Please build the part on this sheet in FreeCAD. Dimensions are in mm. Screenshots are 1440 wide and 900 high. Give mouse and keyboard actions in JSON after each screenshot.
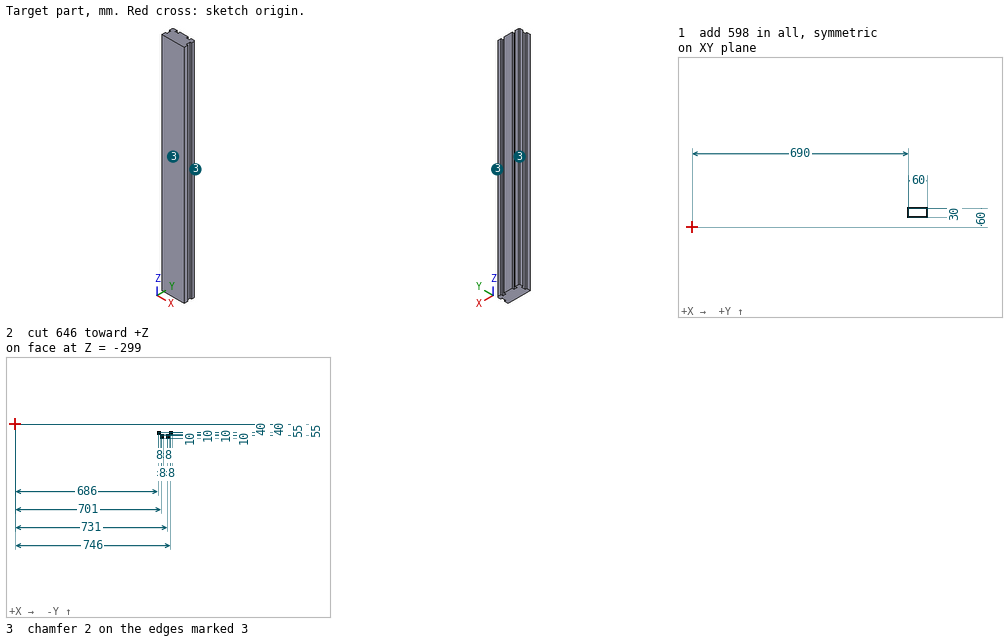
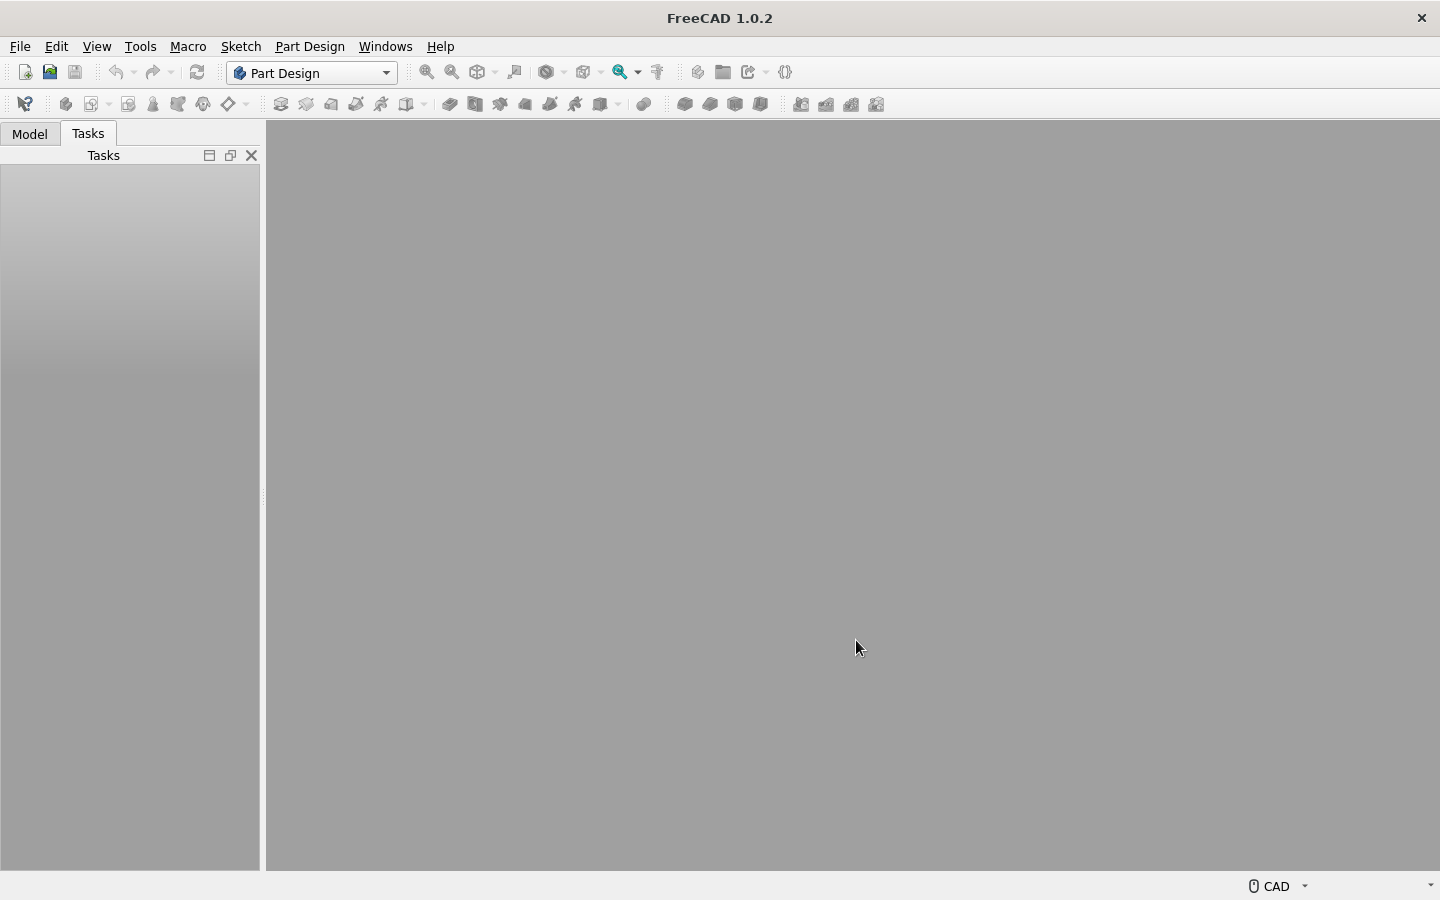
{"action": "left_click", "coordinate": [25, 72]}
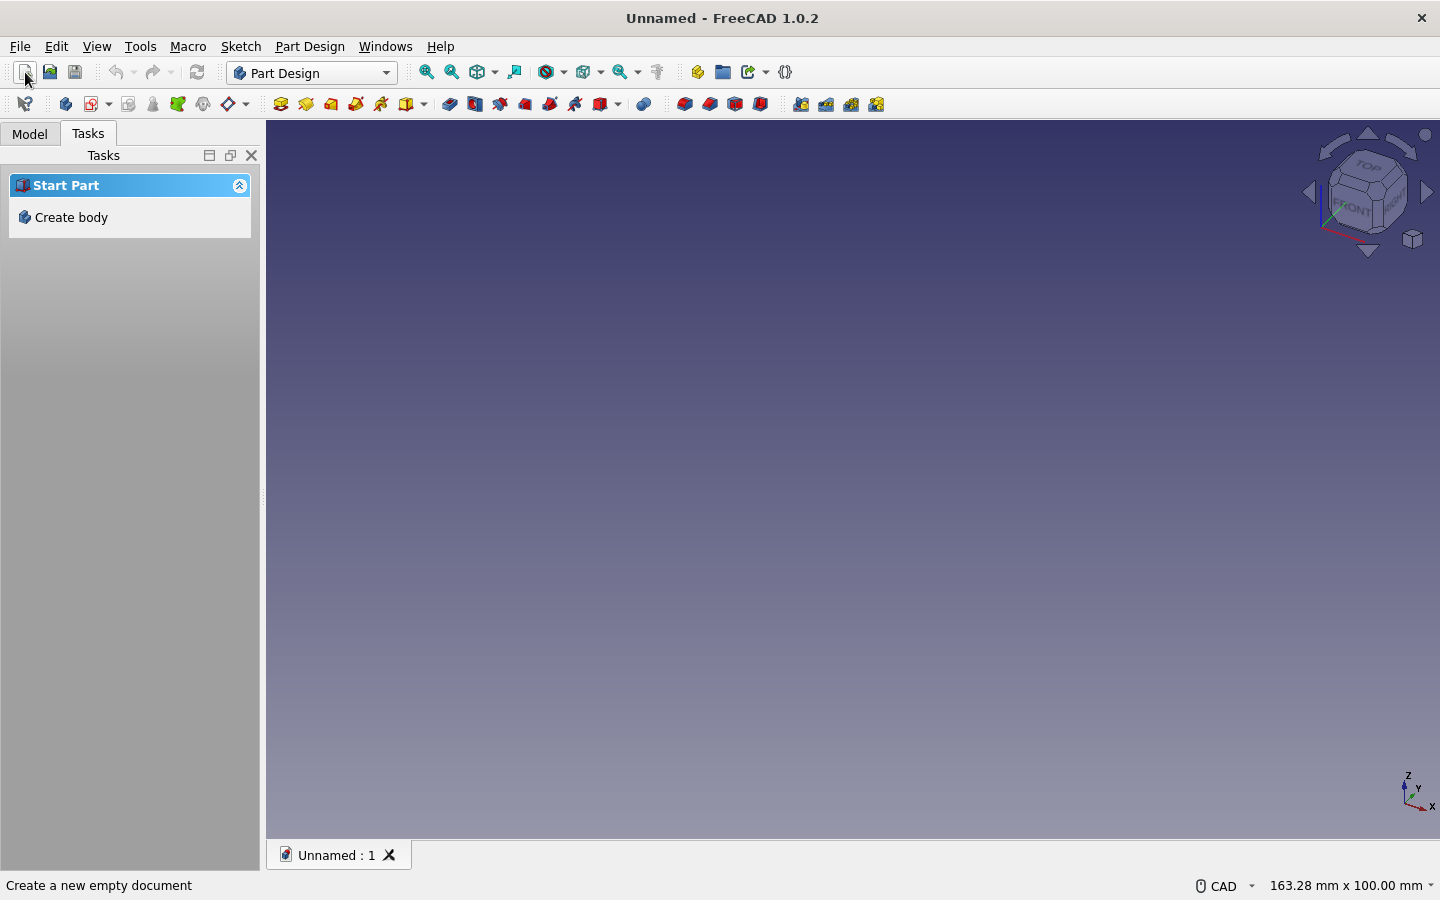
{"action": "left_click", "coordinate": [90, 104]}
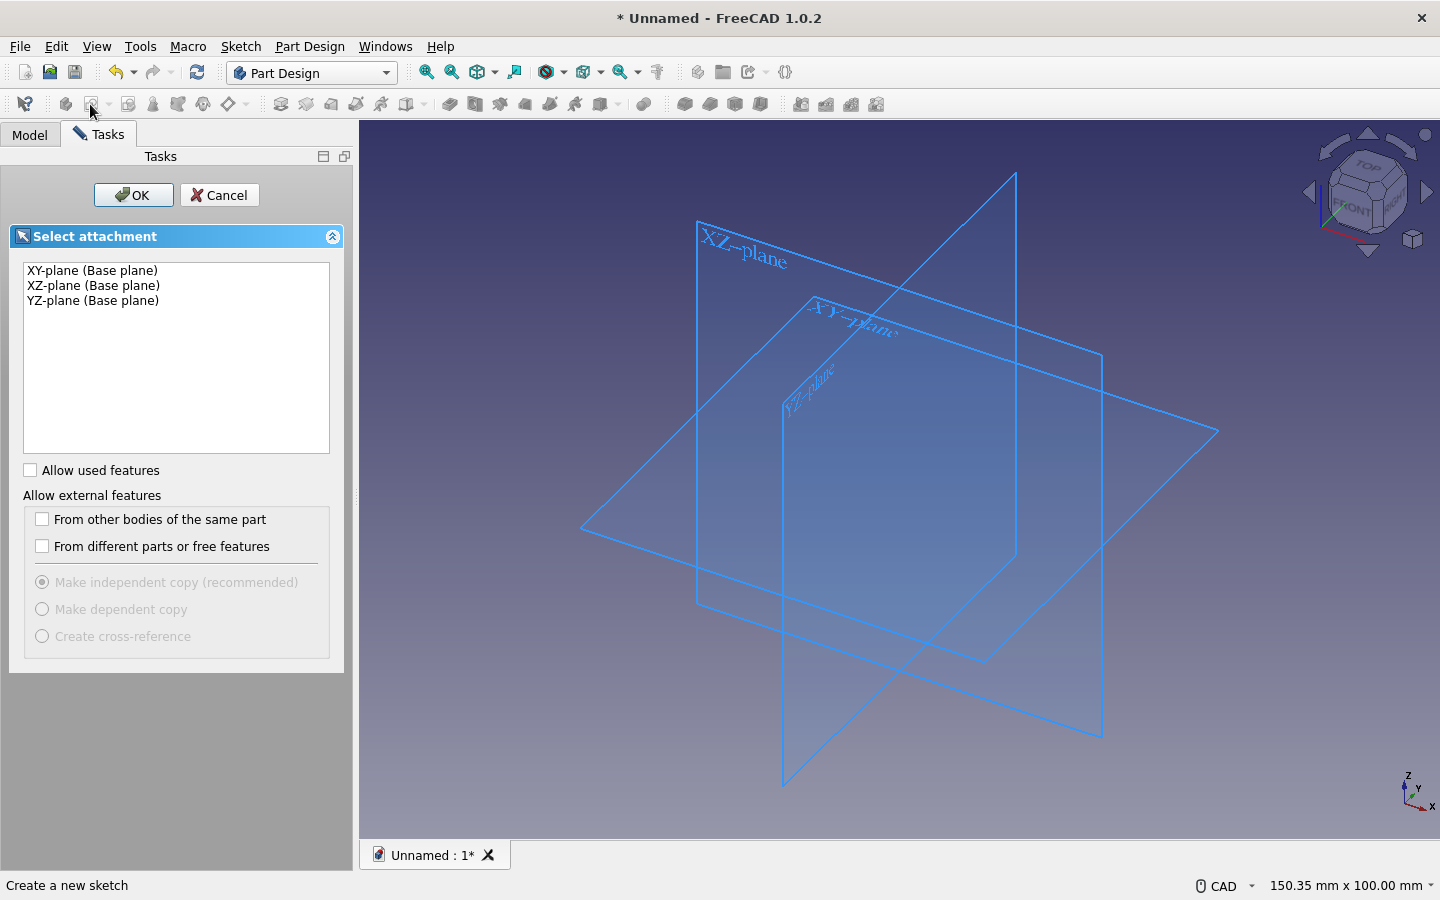
{"action": "left_click", "coordinate": [84, 270]}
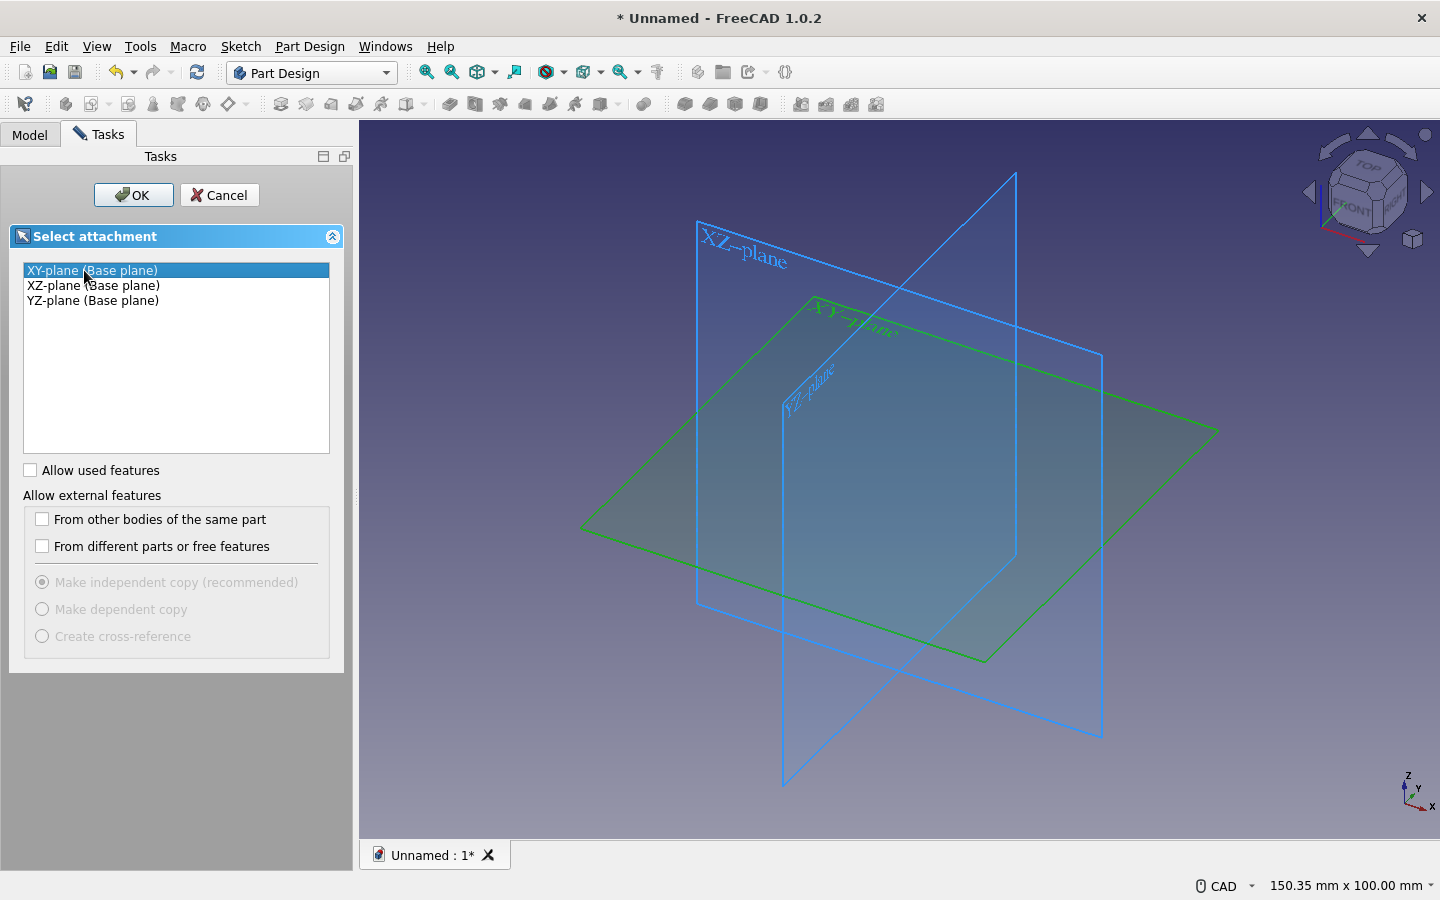
{"action": "left_click", "coordinate": [134, 195]}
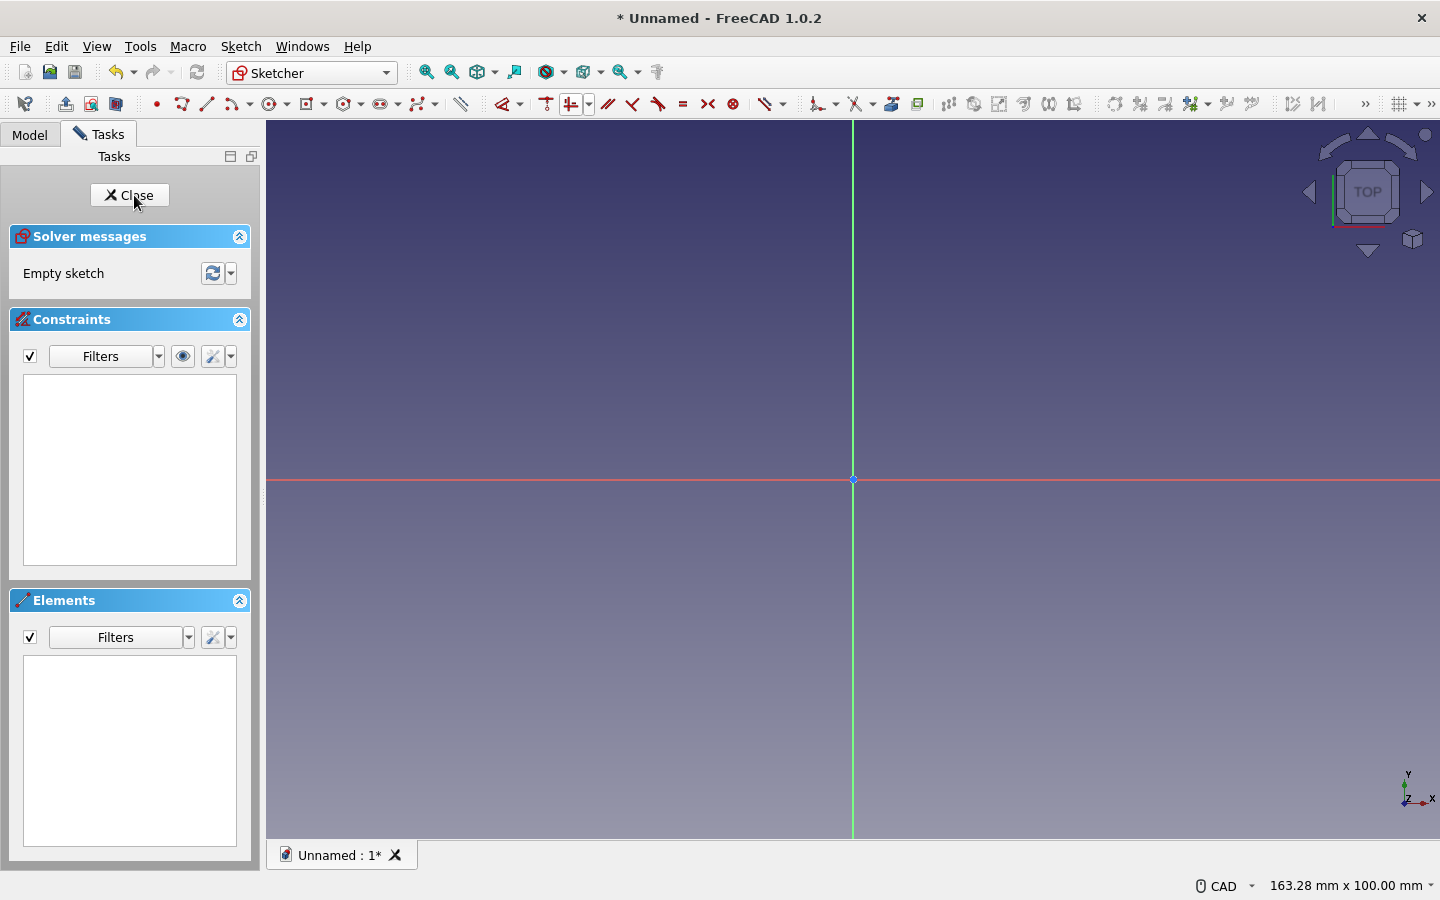
{"action": "scroll", "coordinate": [784, 480], "scroll_direction": "down", "scroll_amount": 5}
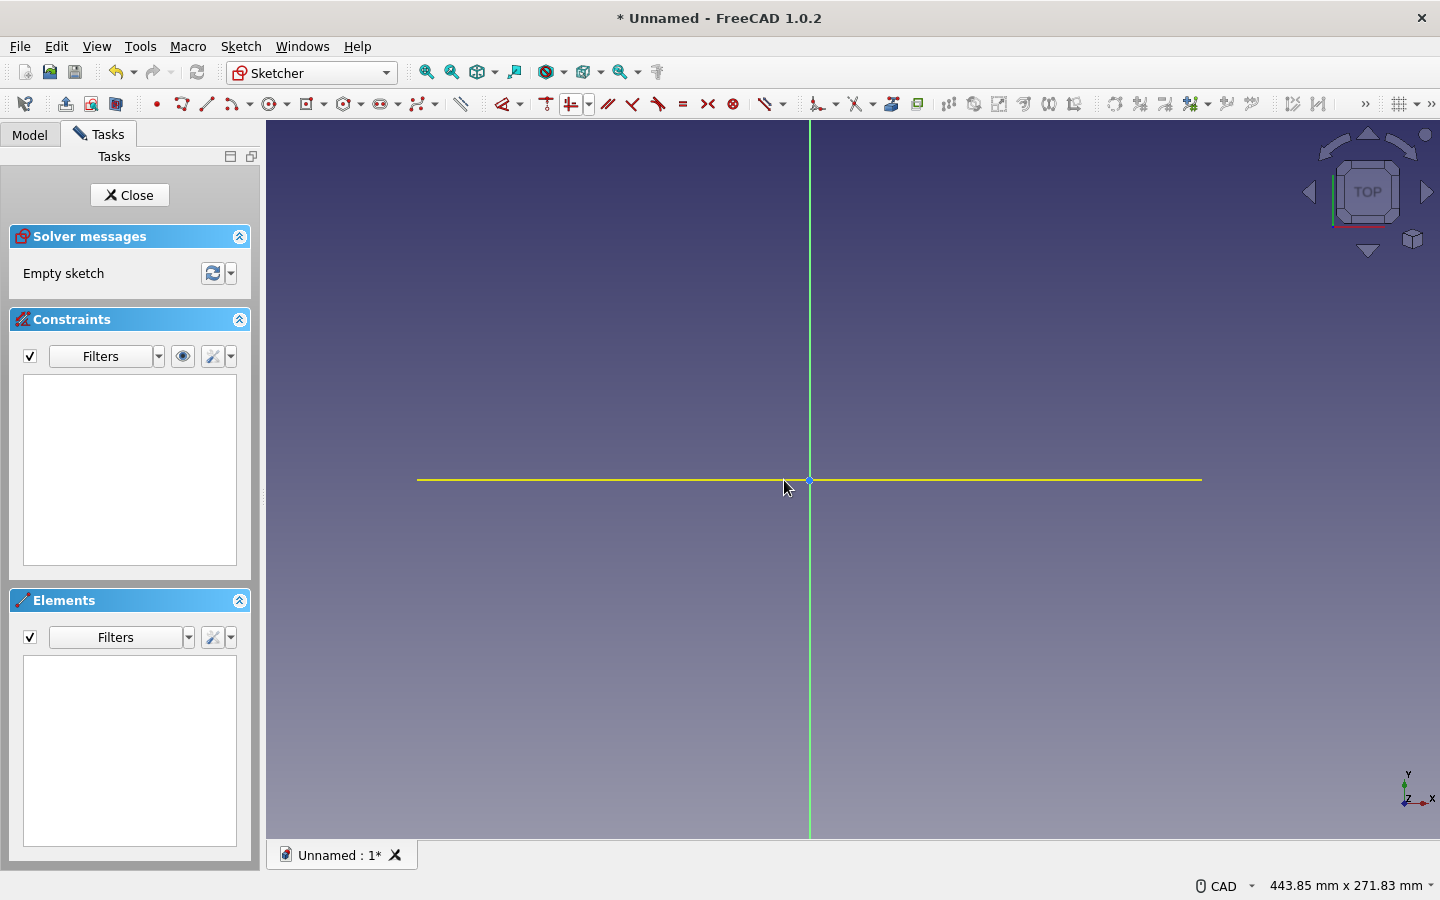
{"action": "scroll", "coordinate": [784, 480], "scroll_direction": "down", "scroll_amount": 5}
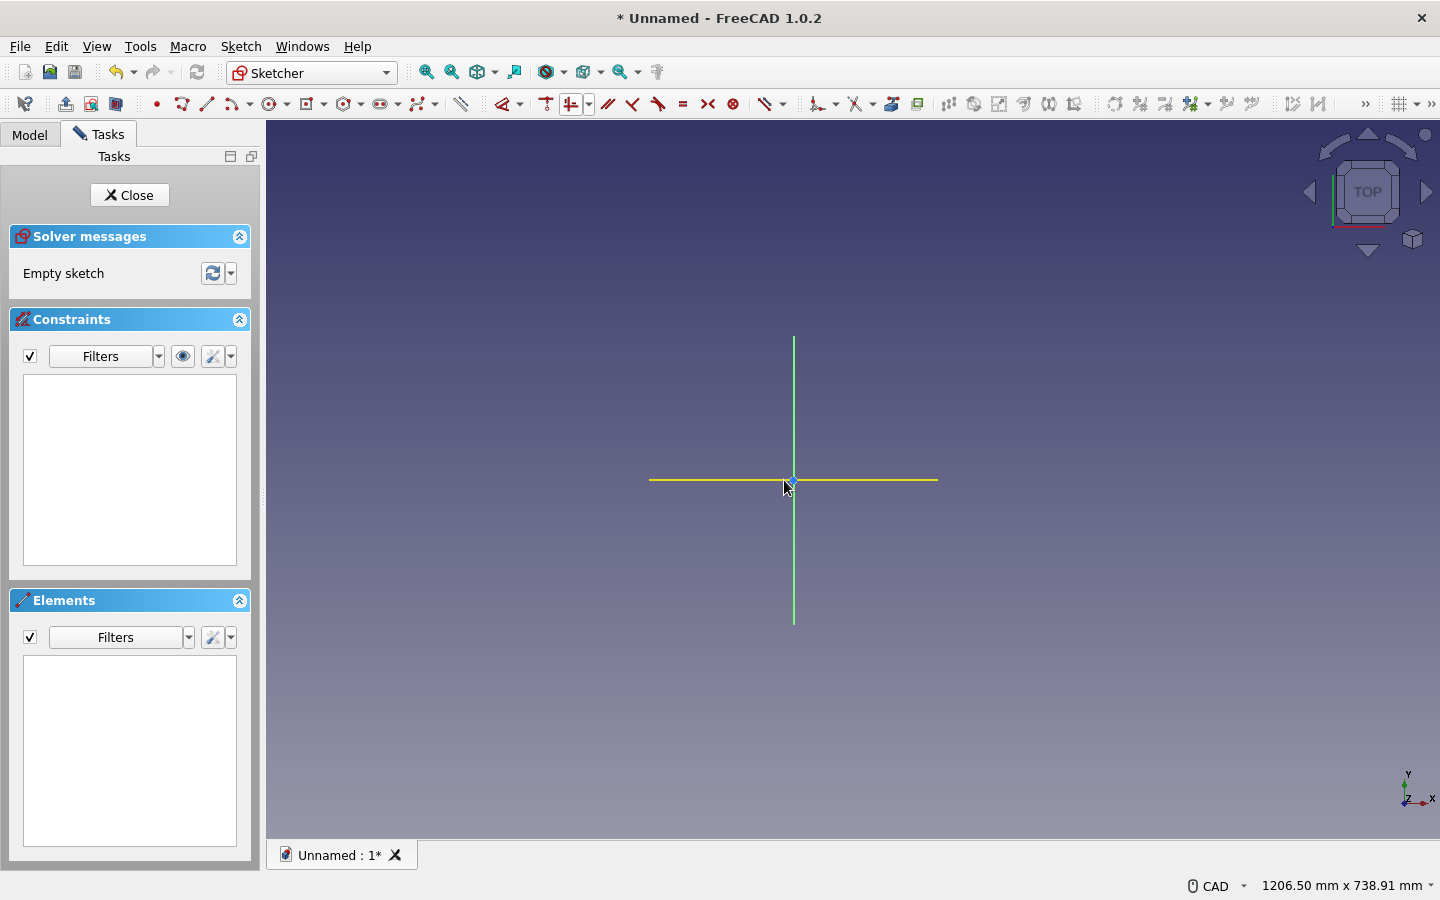
{"action": "scroll", "coordinate": [784, 480], "scroll_direction": "down", "scroll_amount": 5}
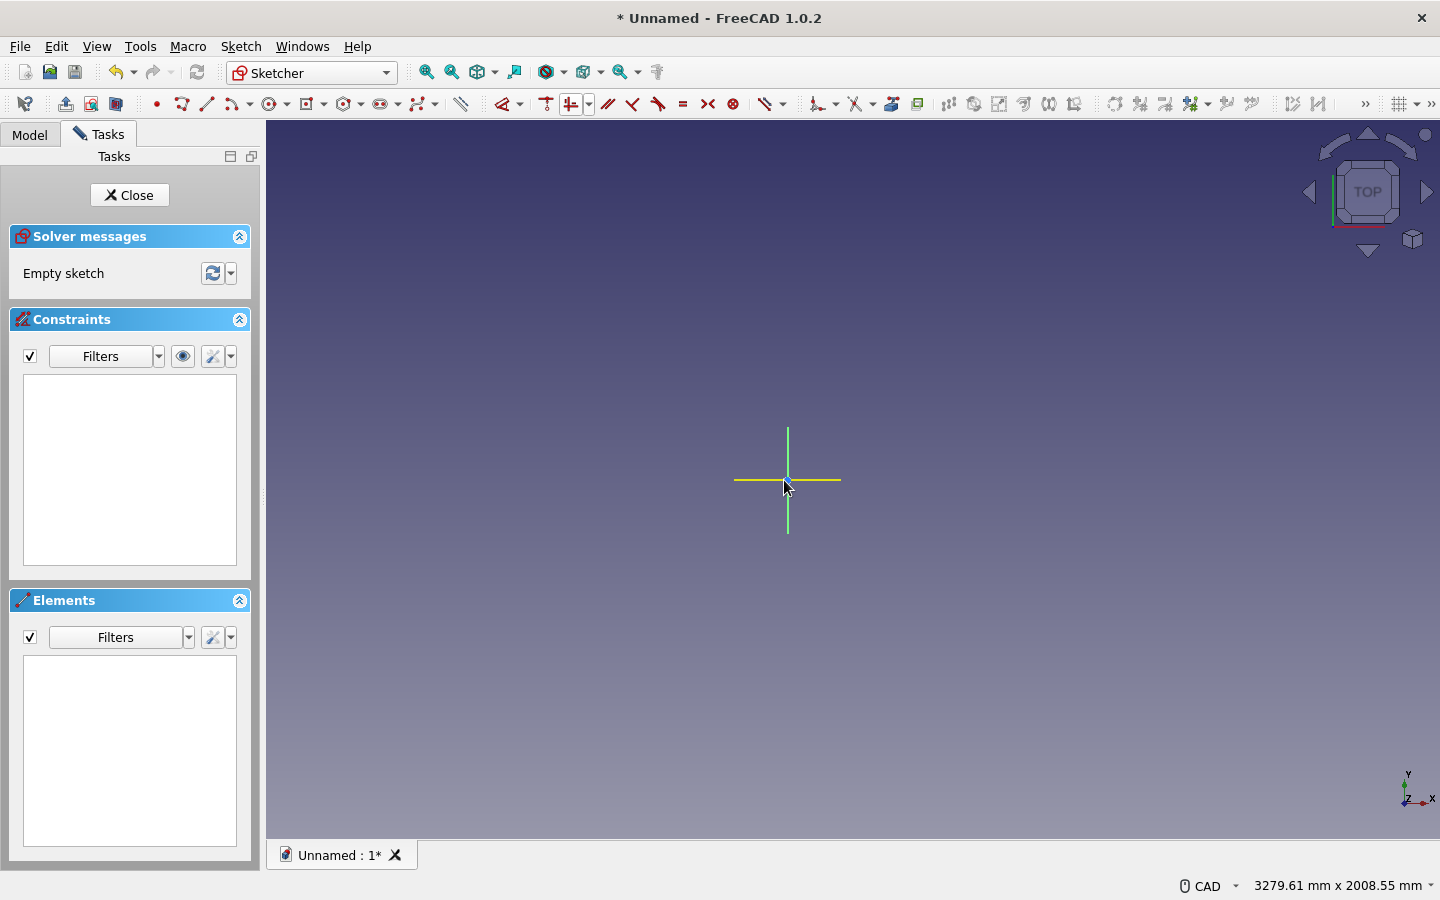
{"action": "scroll", "coordinate": [1059, 464], "scroll_direction": "up", "scroll_amount": 15}